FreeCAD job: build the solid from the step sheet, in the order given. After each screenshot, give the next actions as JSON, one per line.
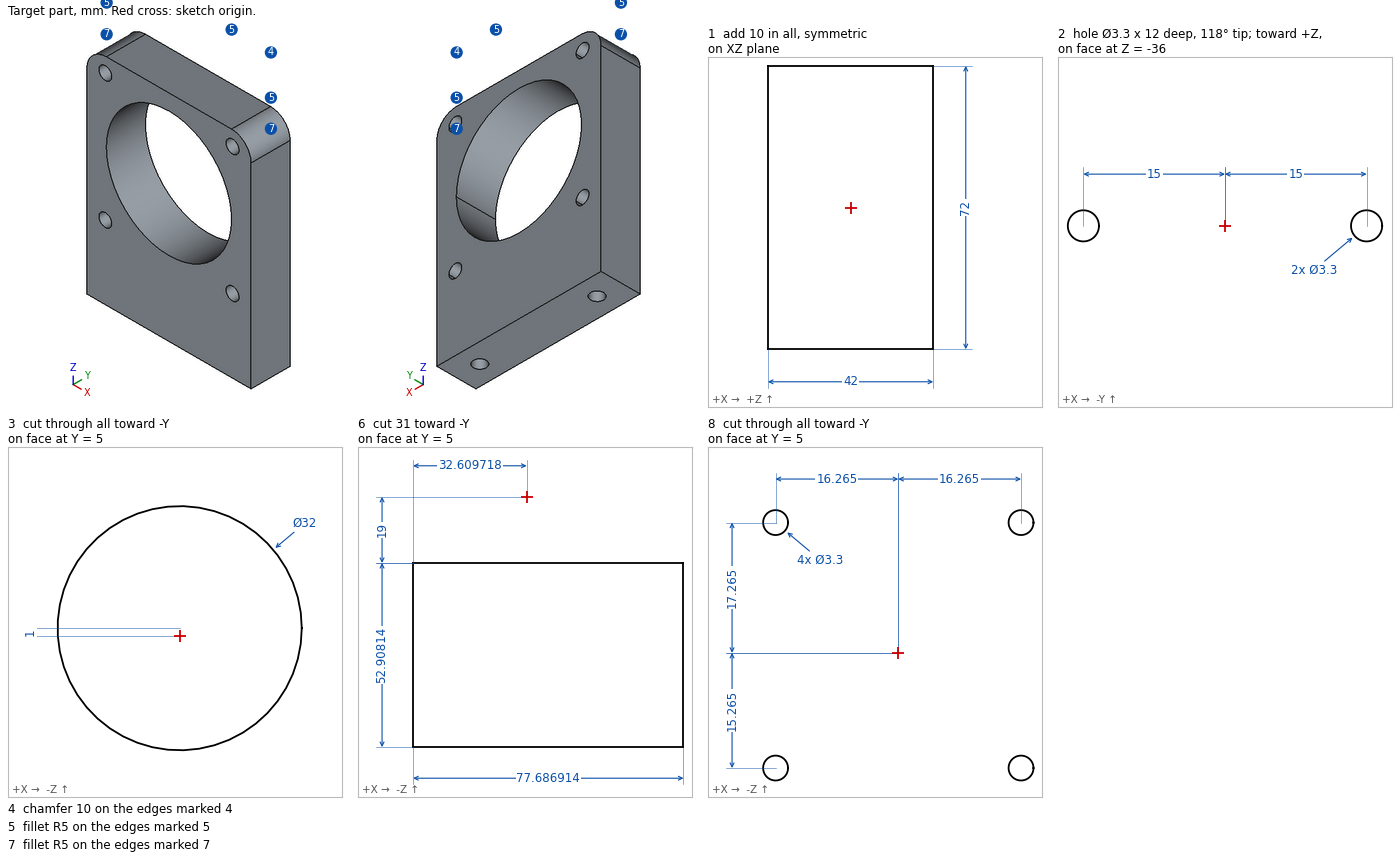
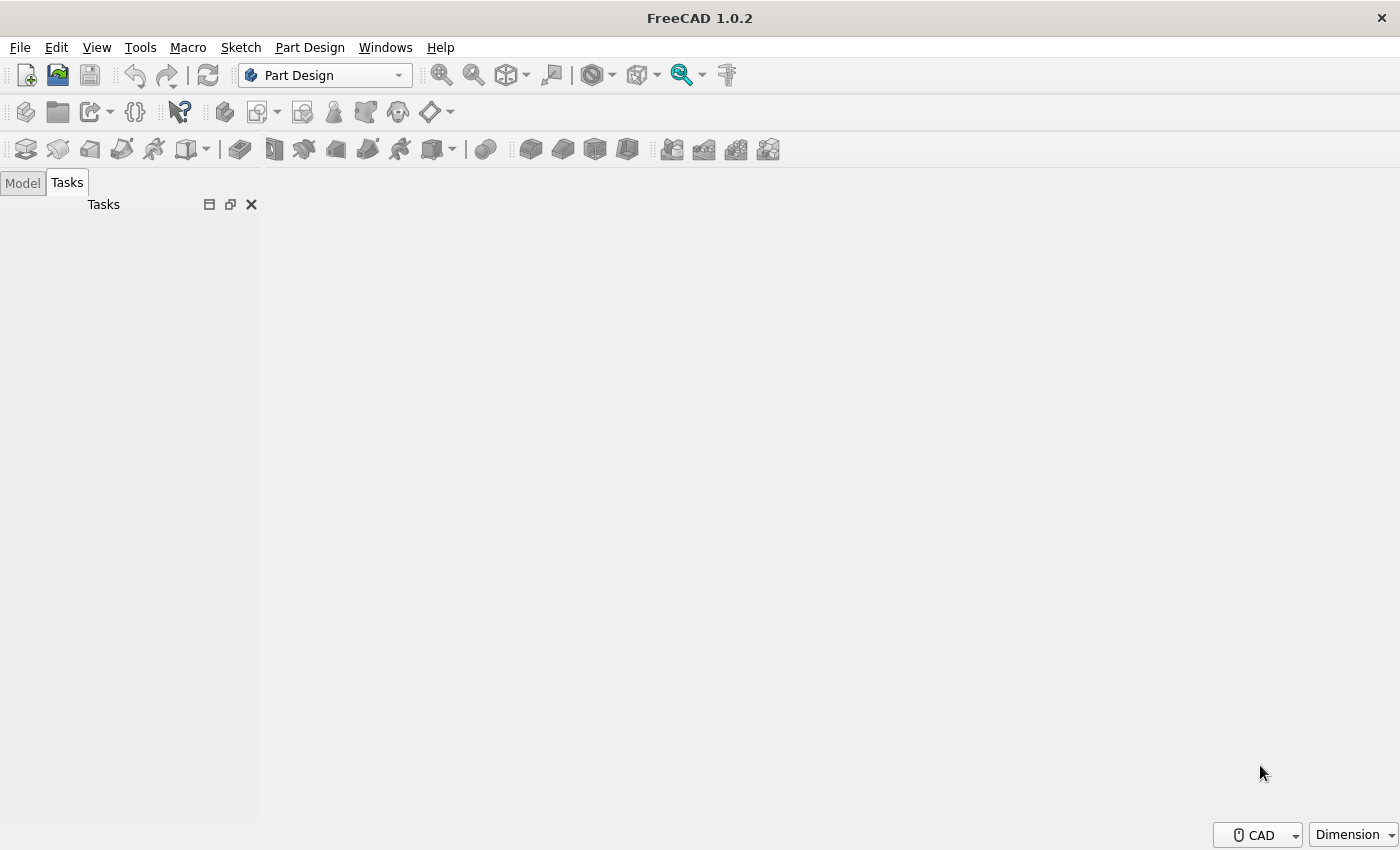
{"action": "left_click", "coordinate": [26, 76]}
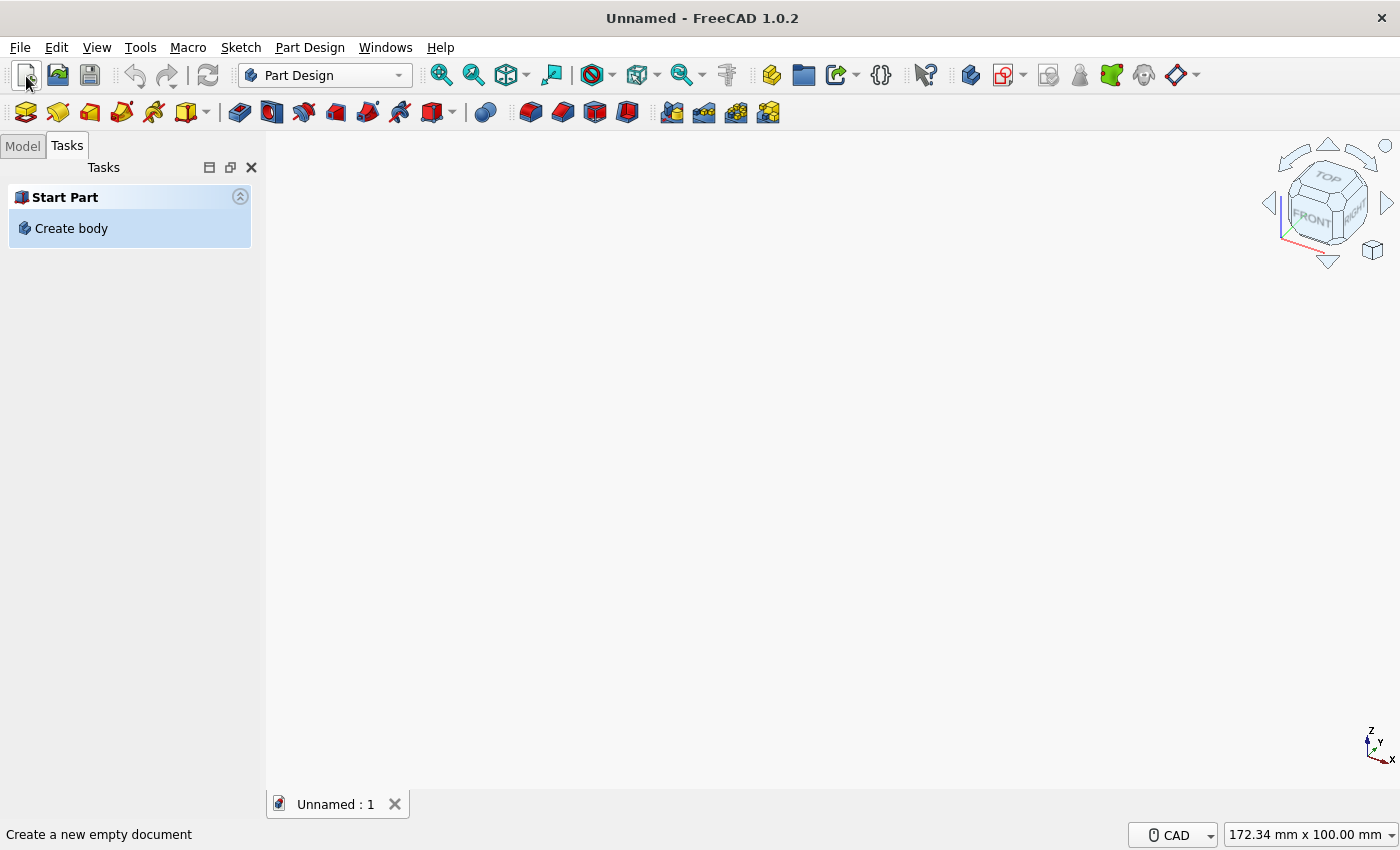
{"action": "left_click", "coordinate": [1004, 76]}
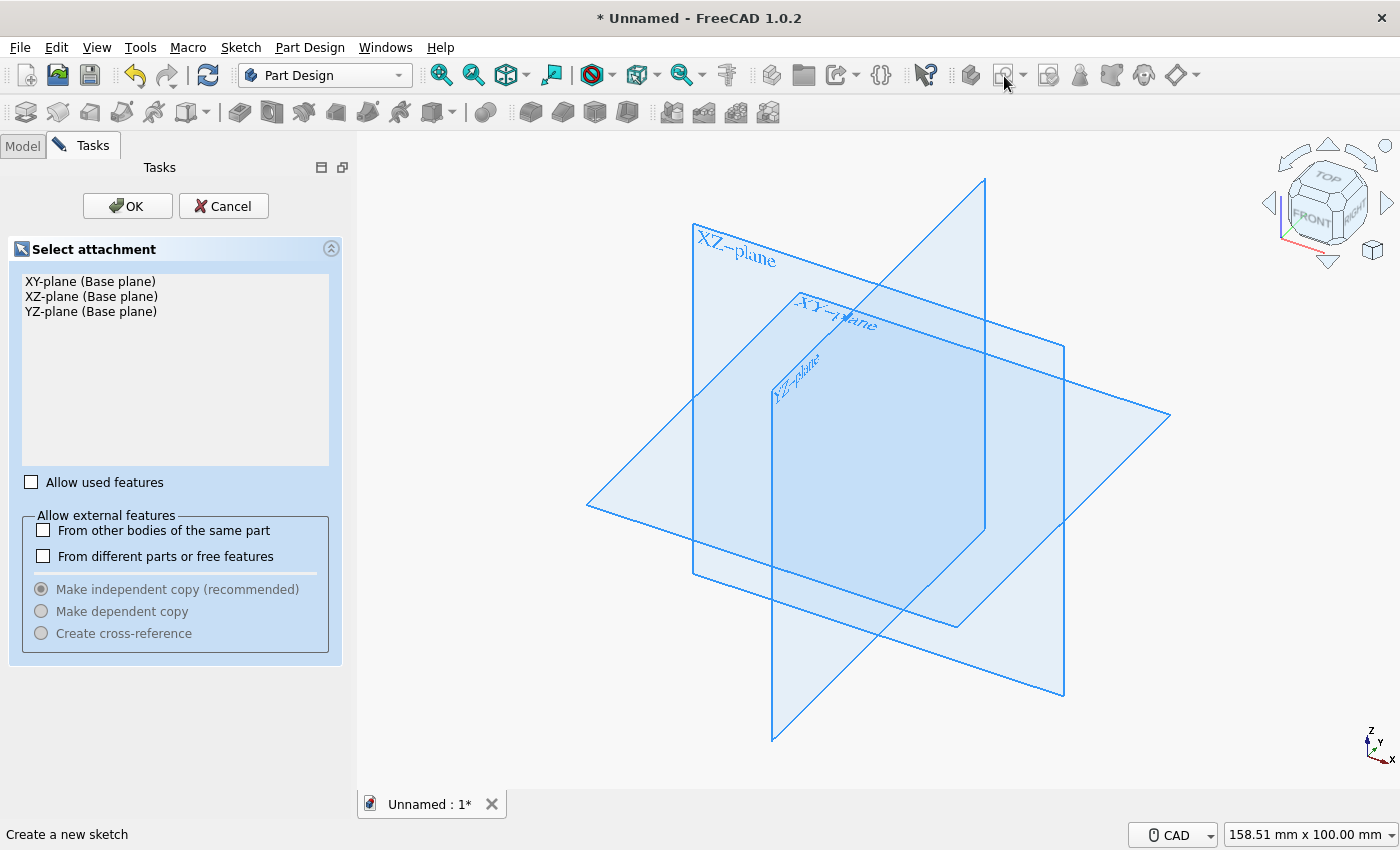
{"action": "left_click", "coordinate": [82, 296]}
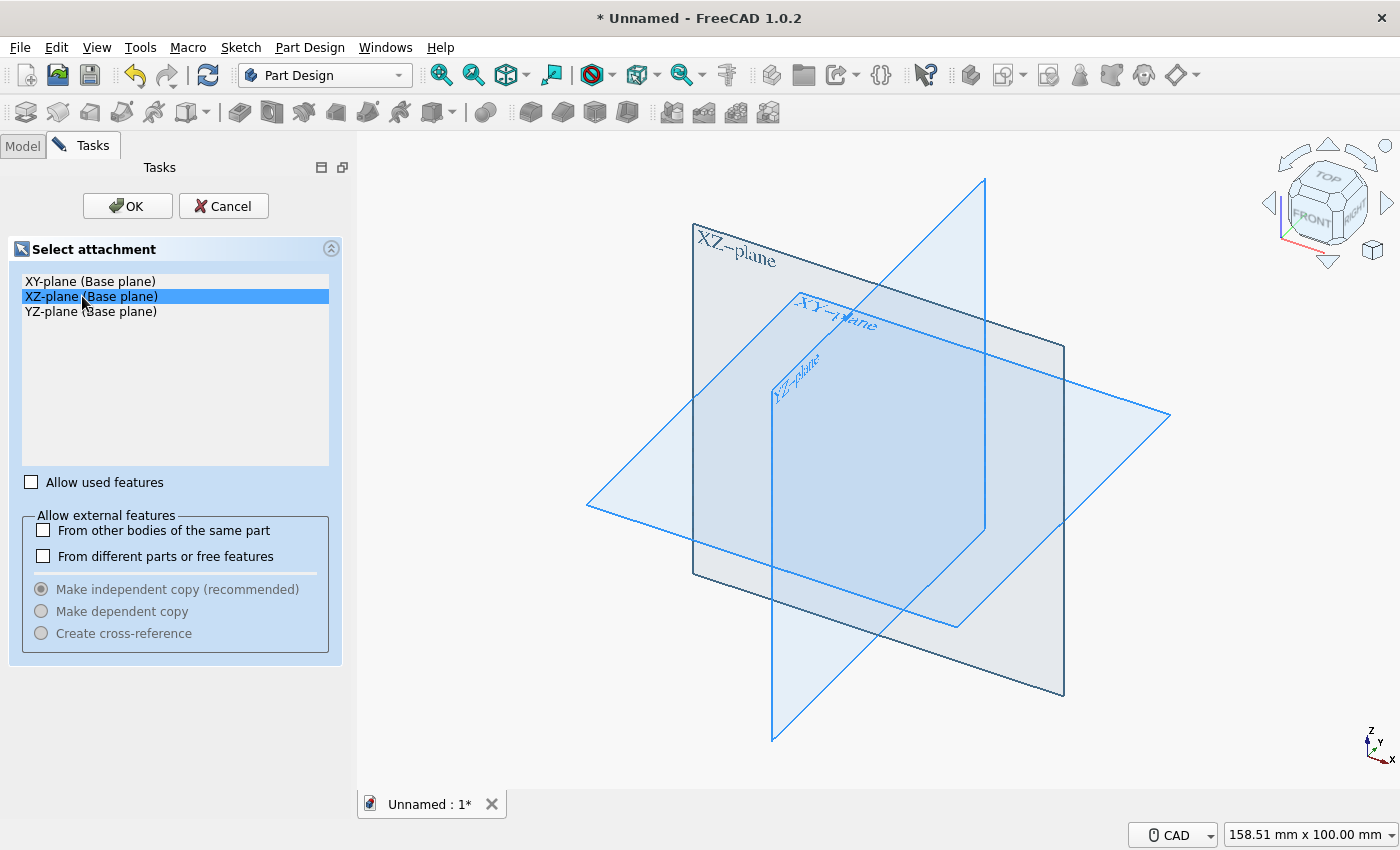
{"action": "left_click", "coordinate": [128, 206]}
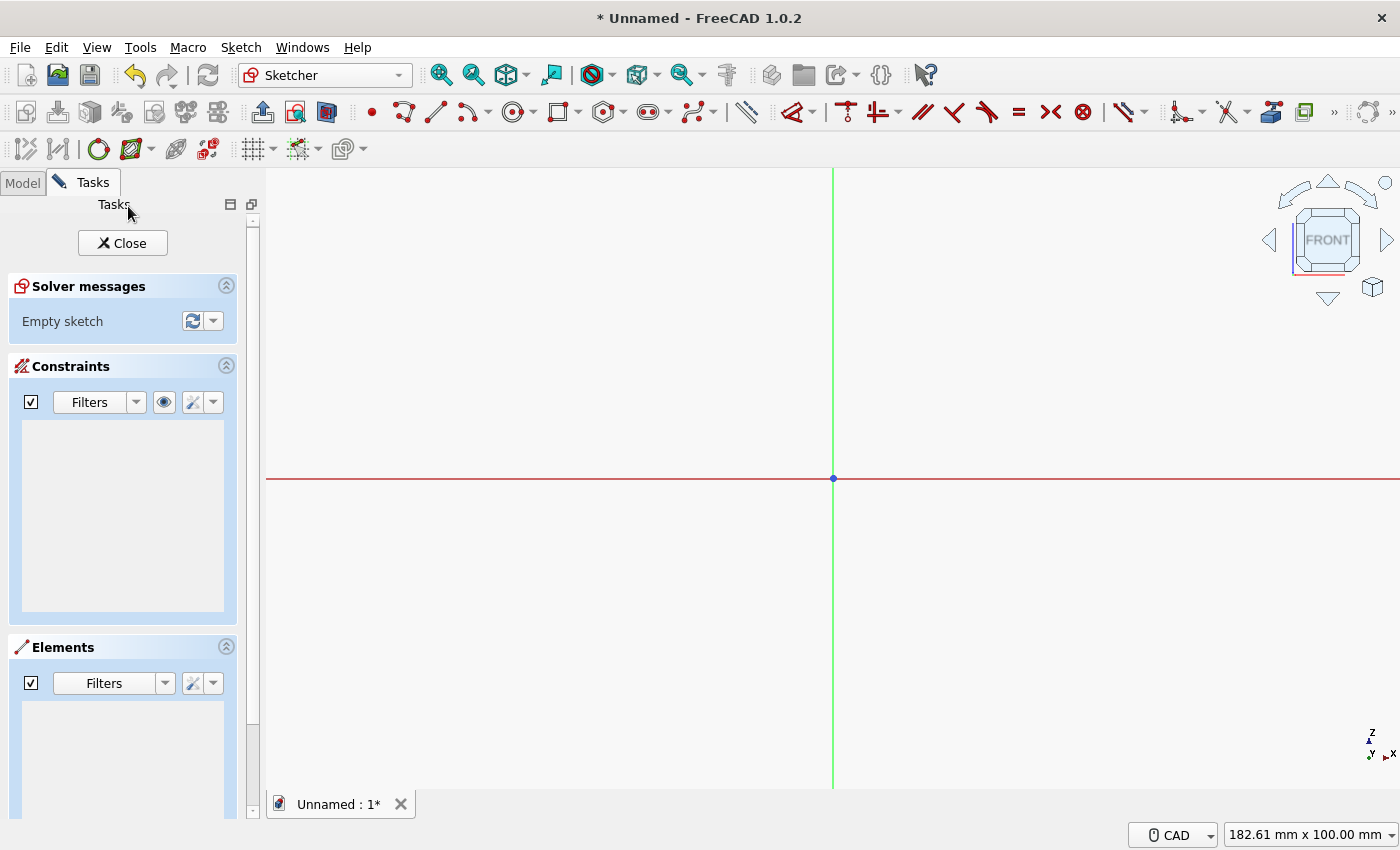
{"action": "left_click", "coordinate": [580, 112]}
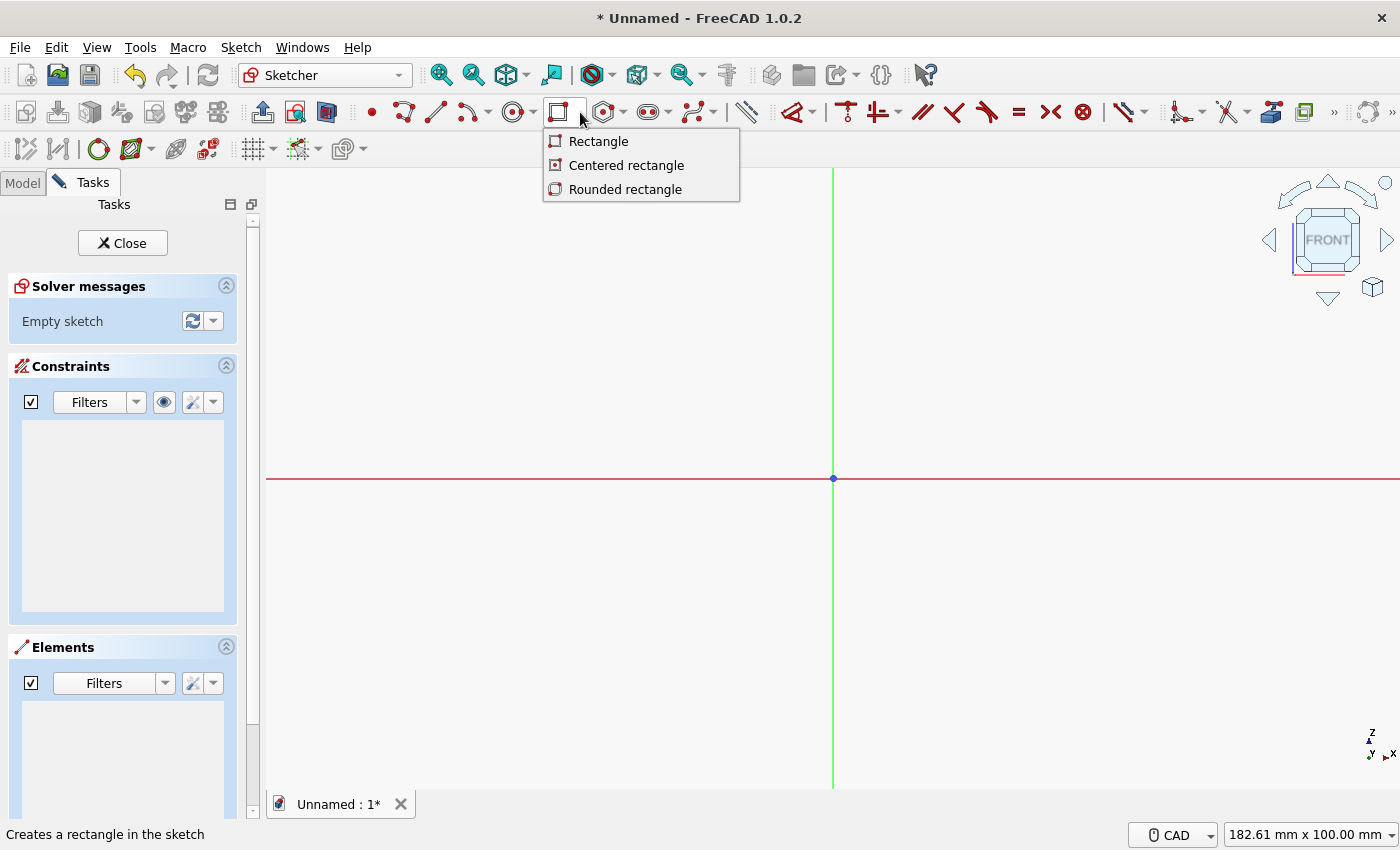
{"action": "left_click", "coordinate": [642, 165]}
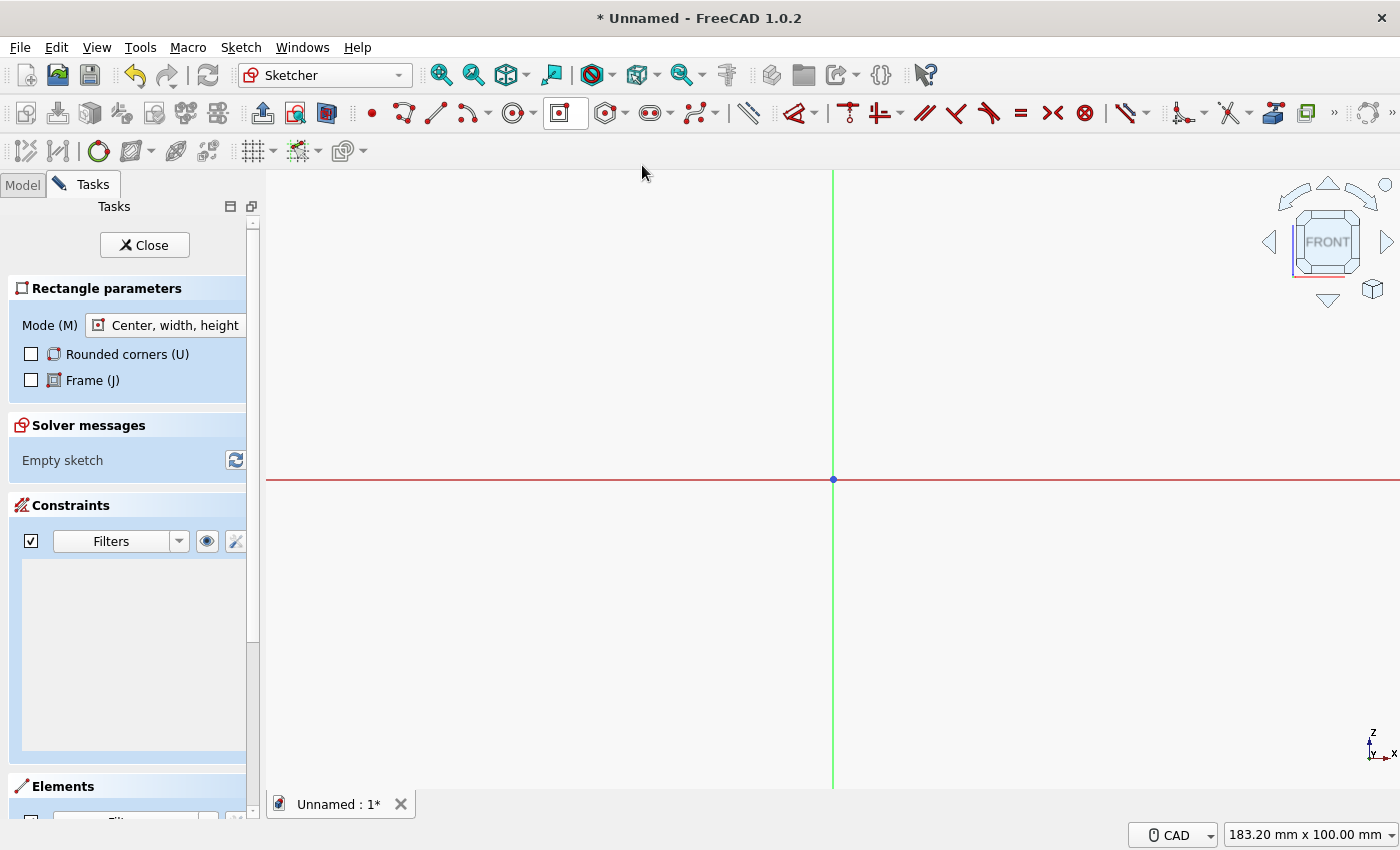
{"action": "left_click", "coordinate": [833, 480]}
{"action": "left_click", "coordinate": [963, 257]}
{"action": "key", "text": "Escape"}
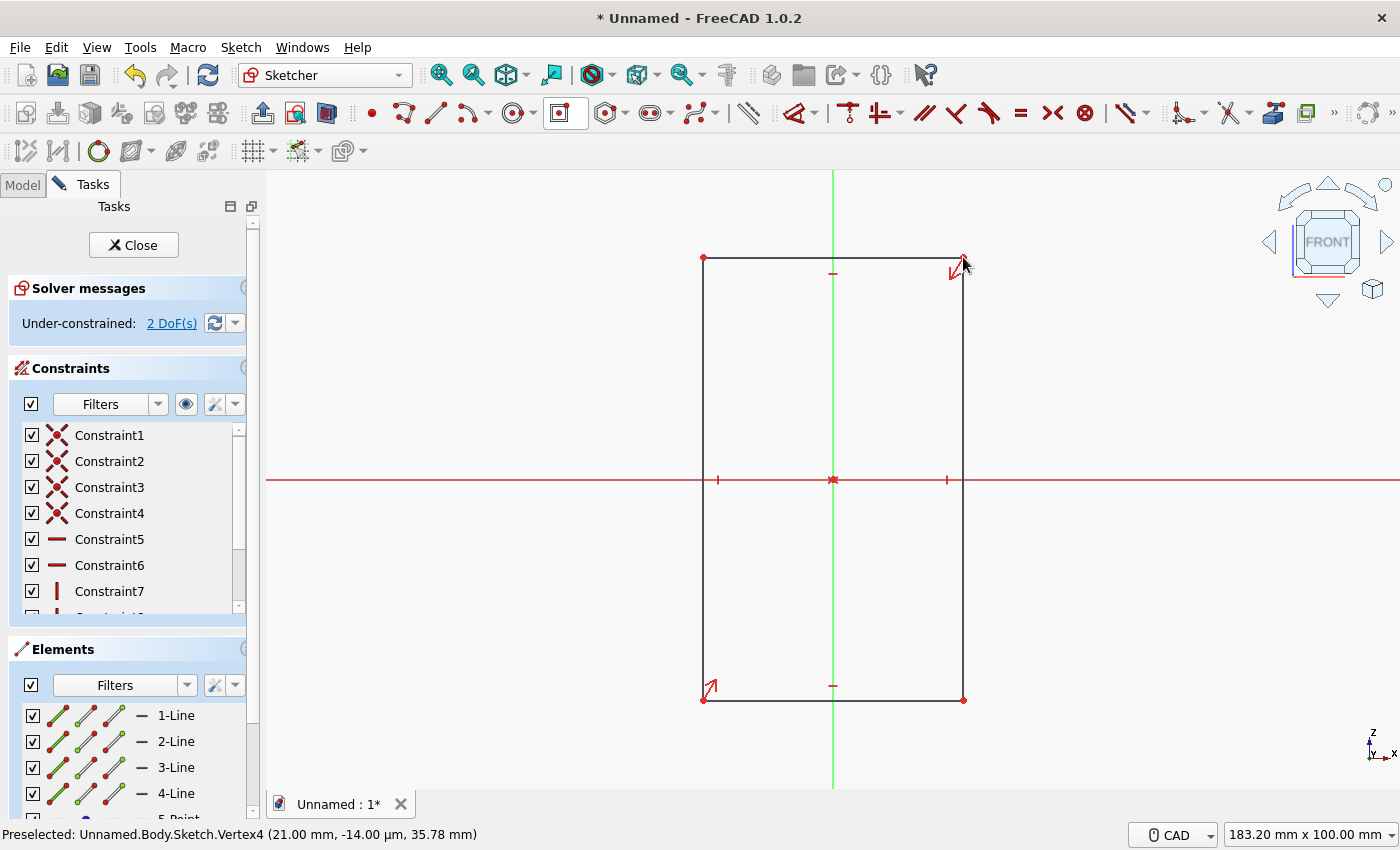
{"action": "left_click", "coordinate": [794, 114]}